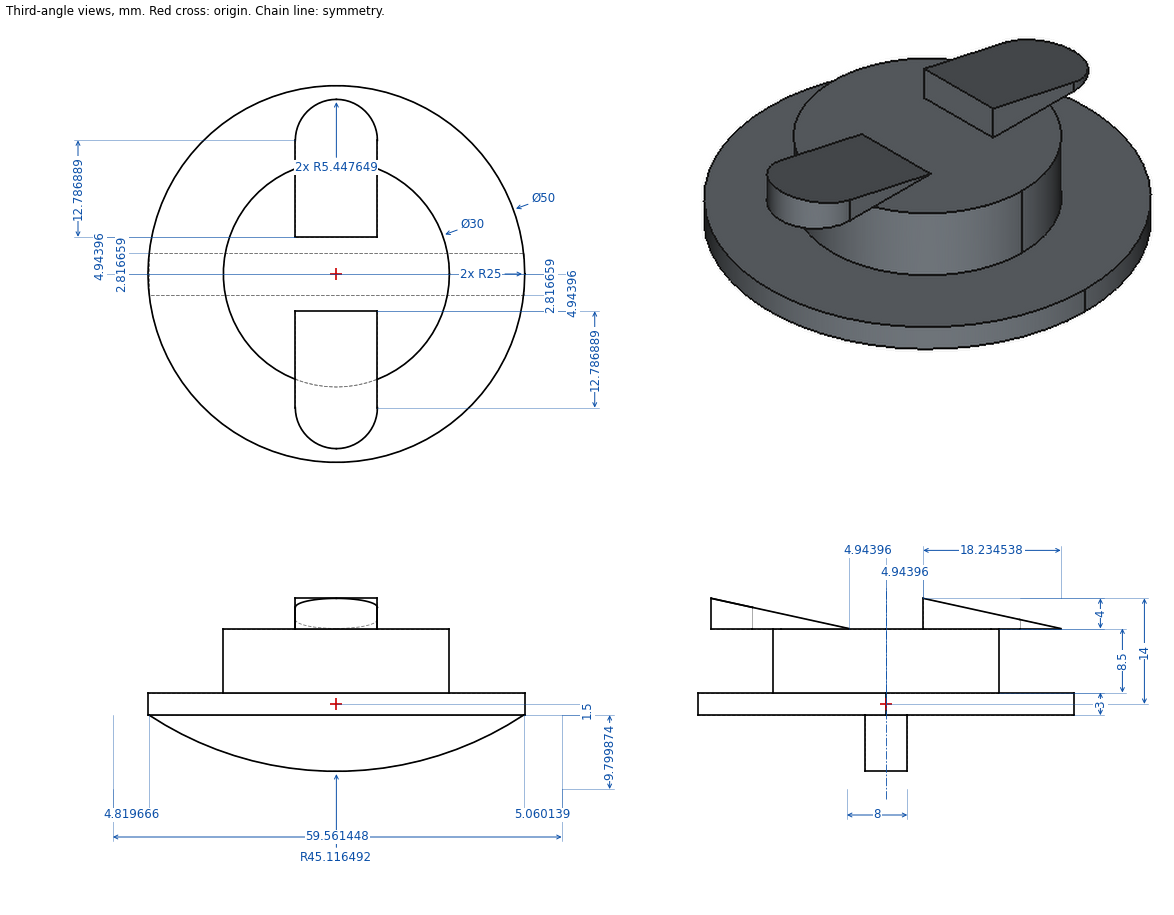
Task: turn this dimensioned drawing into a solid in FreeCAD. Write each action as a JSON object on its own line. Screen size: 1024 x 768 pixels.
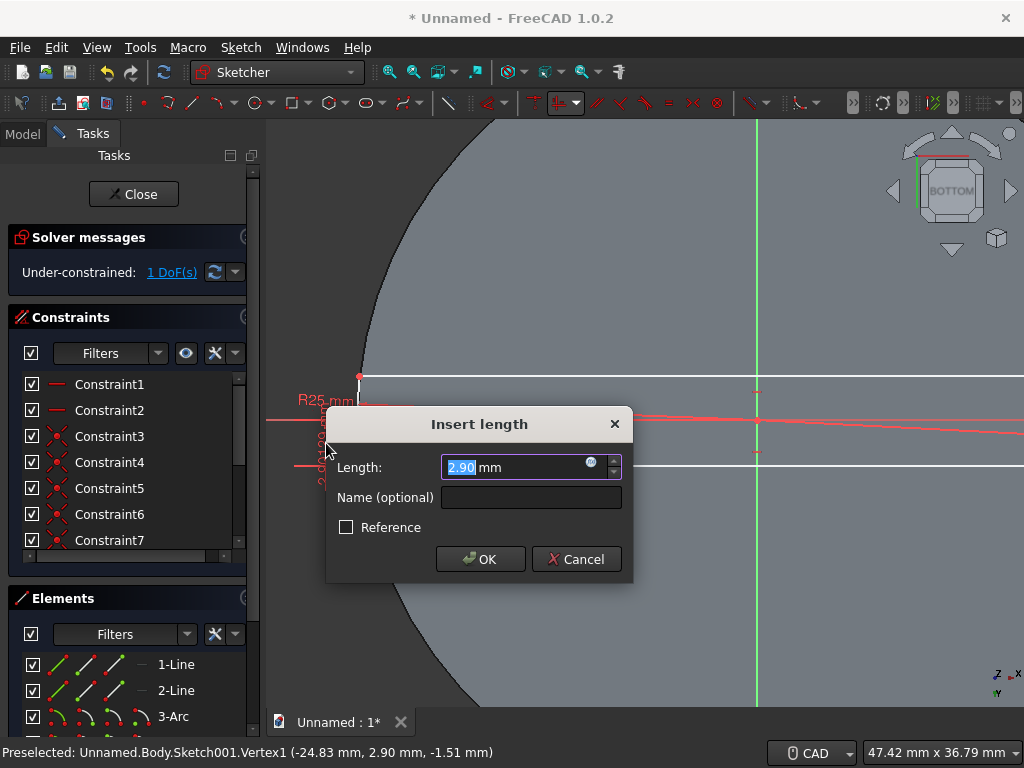
{"action": "type", "text": "2.816659"}
{"action": "key", "text": "Return"}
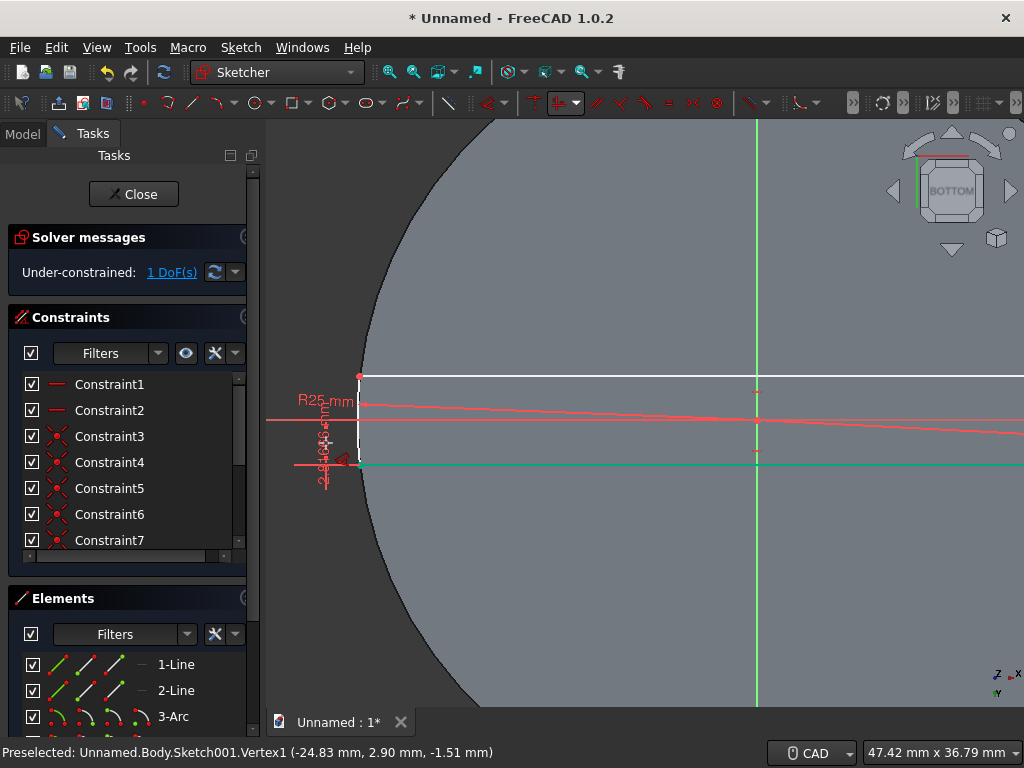
{"action": "scroll", "coordinate": [357, 404], "scroll_direction": "down", "scroll_amount": 3}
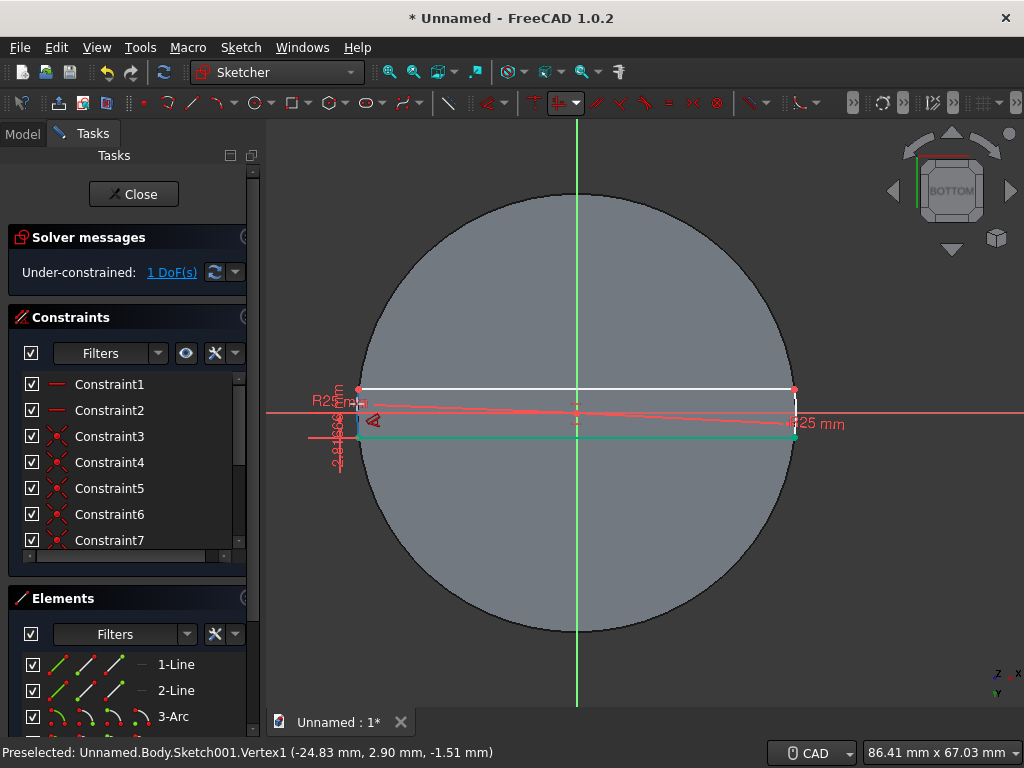
{"action": "scroll", "coordinate": [795, 389], "scroll_direction": "up", "scroll_amount": 3}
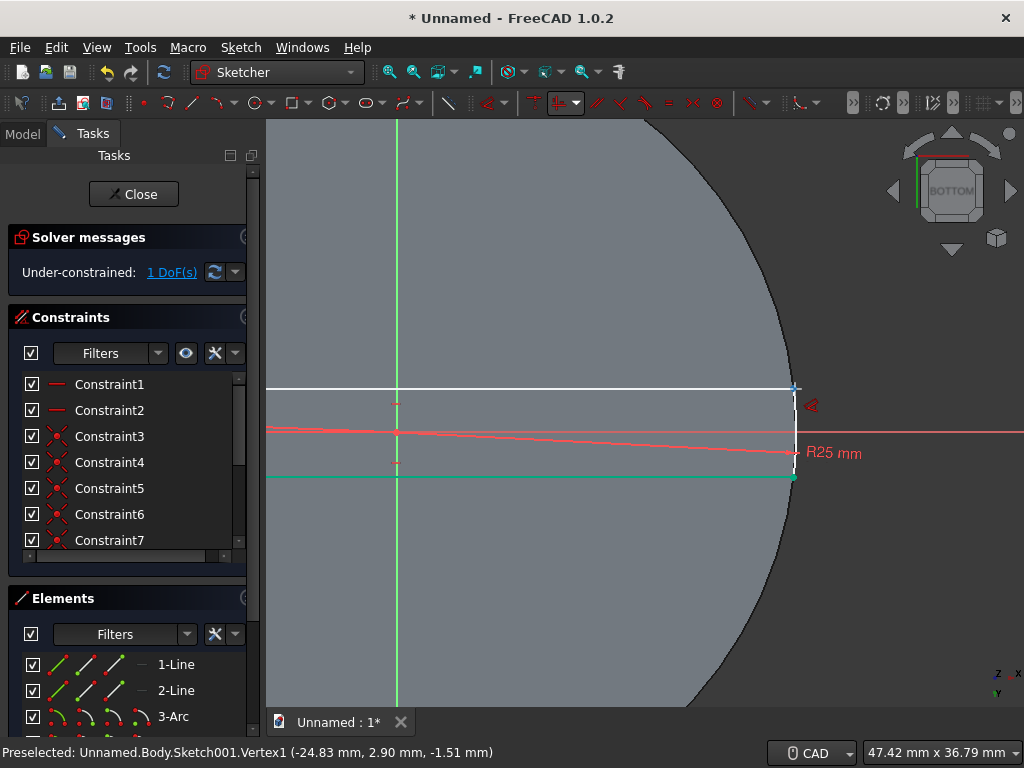
{"action": "left_click", "coordinate": [794, 389]}
{"action": "left_click", "coordinate": [828, 411]}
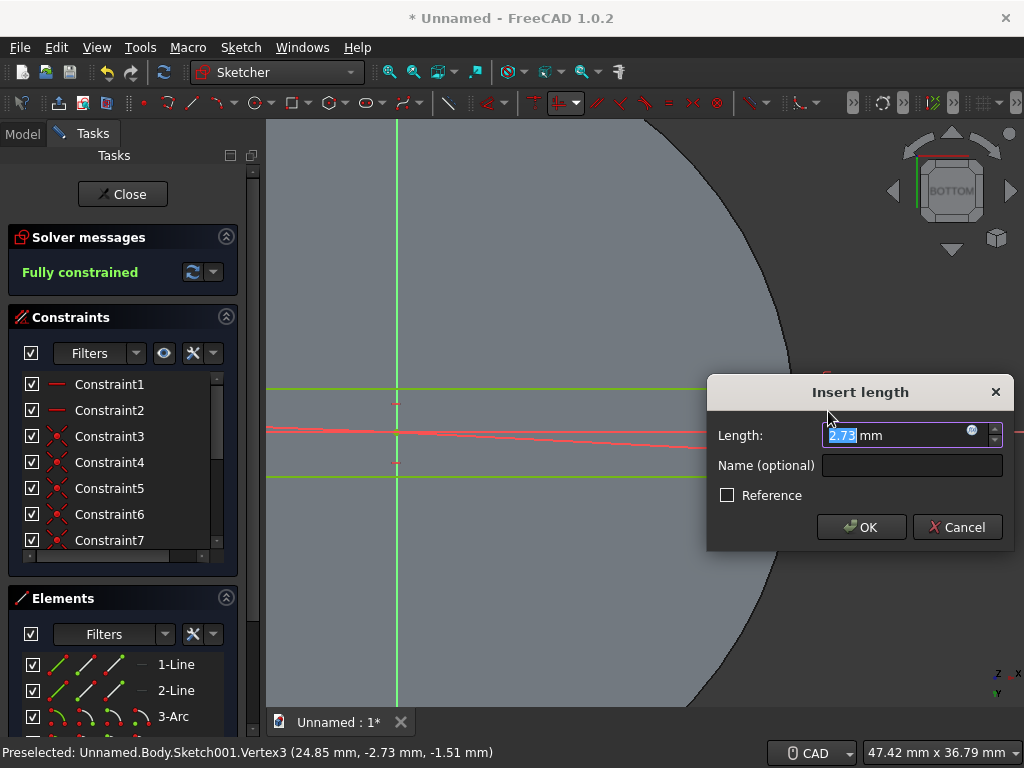
{"action": "type", "text": "2.816659"}
{"action": "key", "text": "Return"}
{"action": "key", "text": "Escape"}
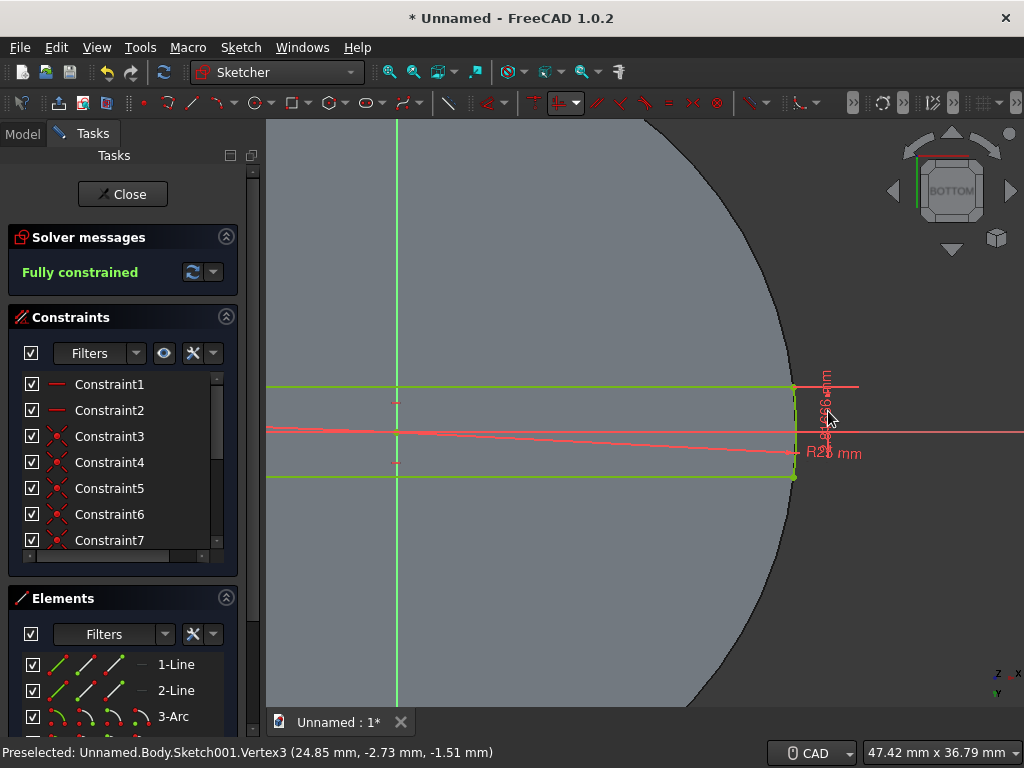
{"action": "left_click", "coordinate": [123, 194]}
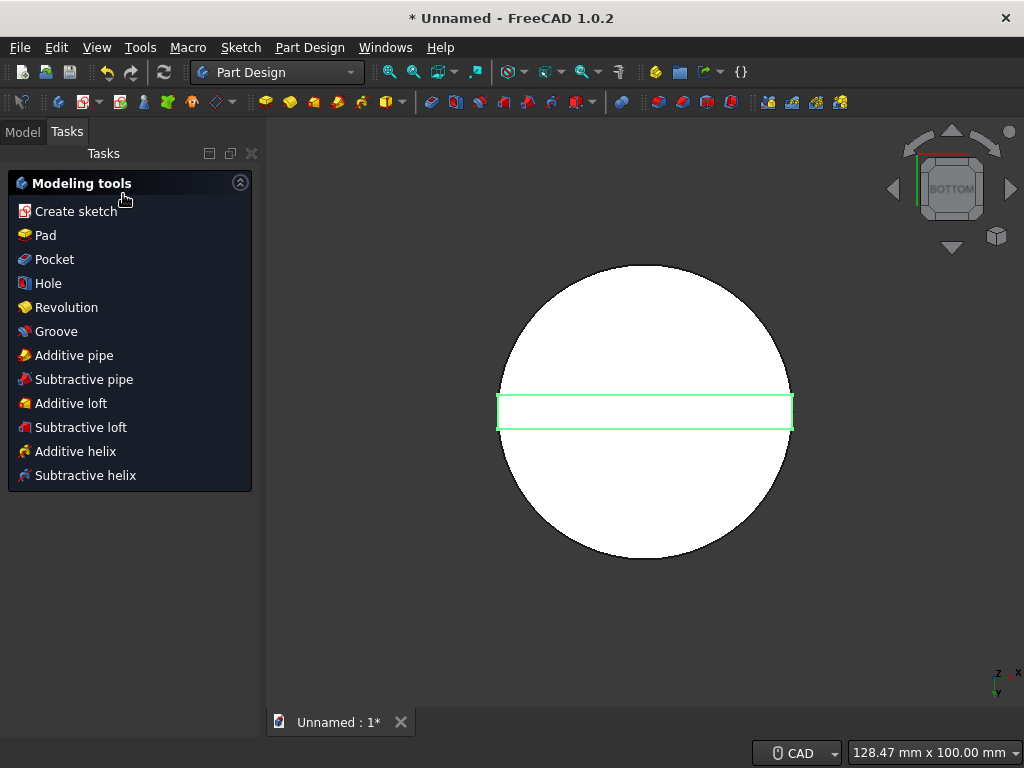
{"action": "left_click", "coordinate": [266, 102]}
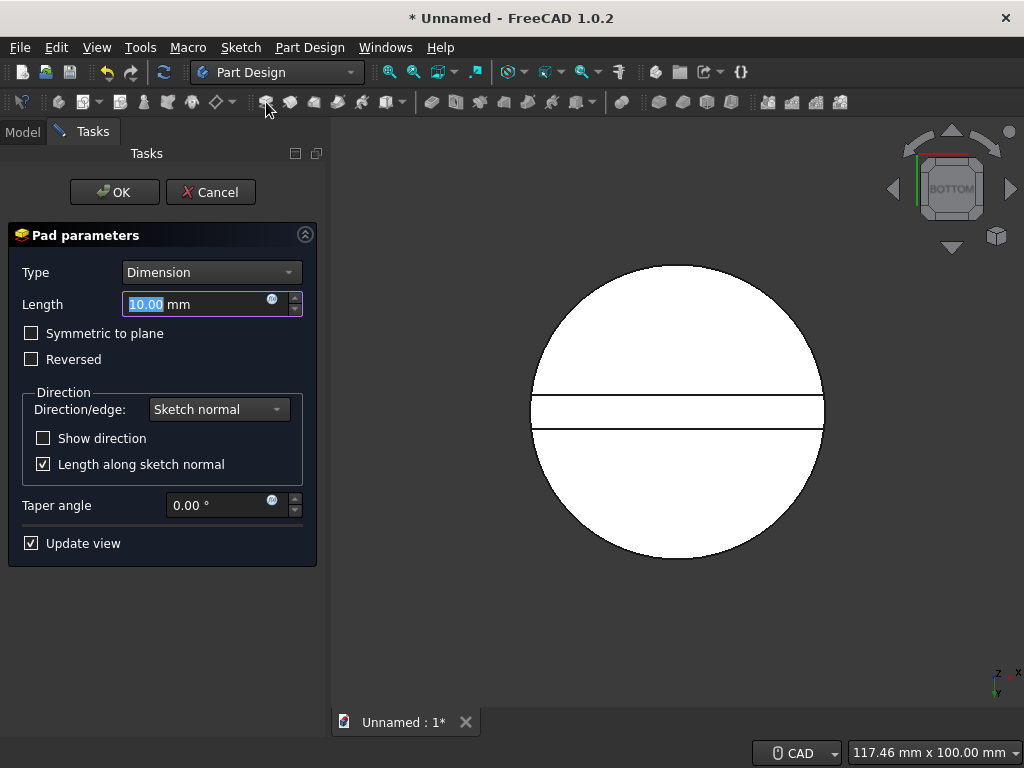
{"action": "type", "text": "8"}
{"action": "key", "text": "Tab"}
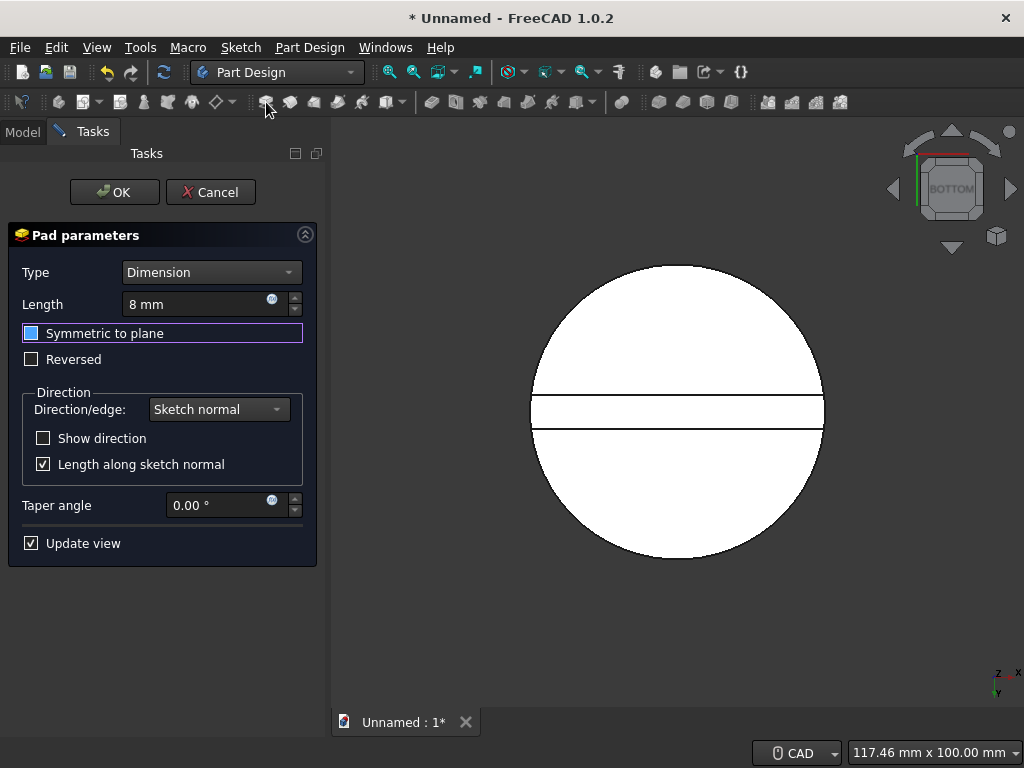
{"action": "left_click", "coordinate": [115, 192]}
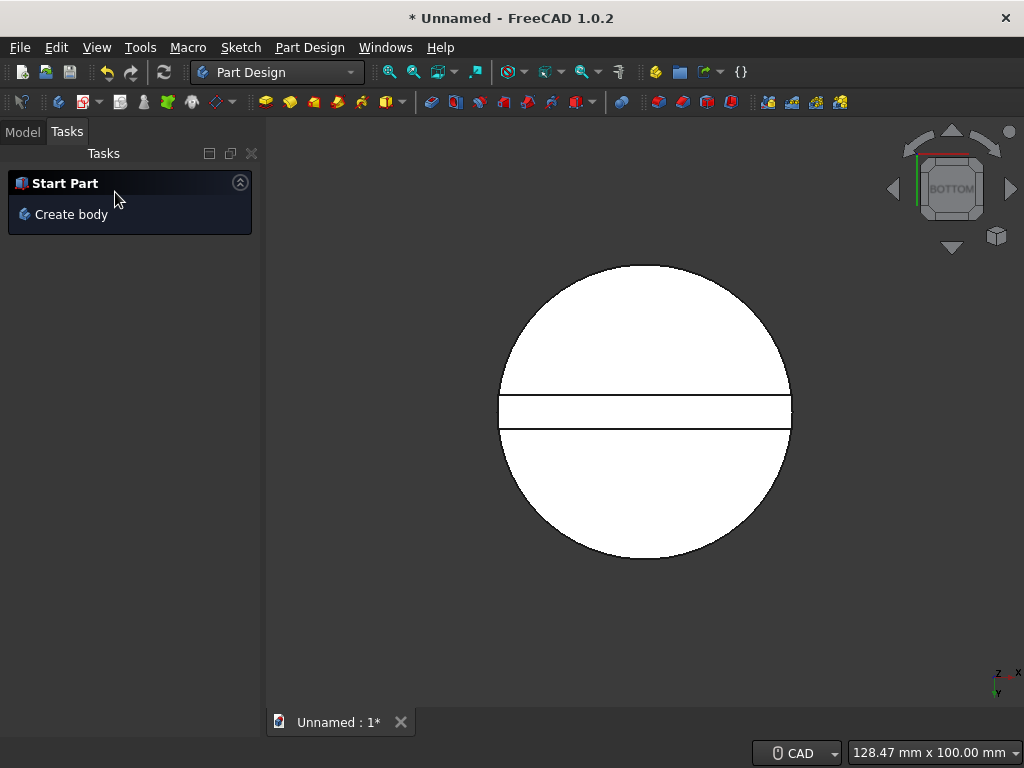
{"action": "key", "text": "4"}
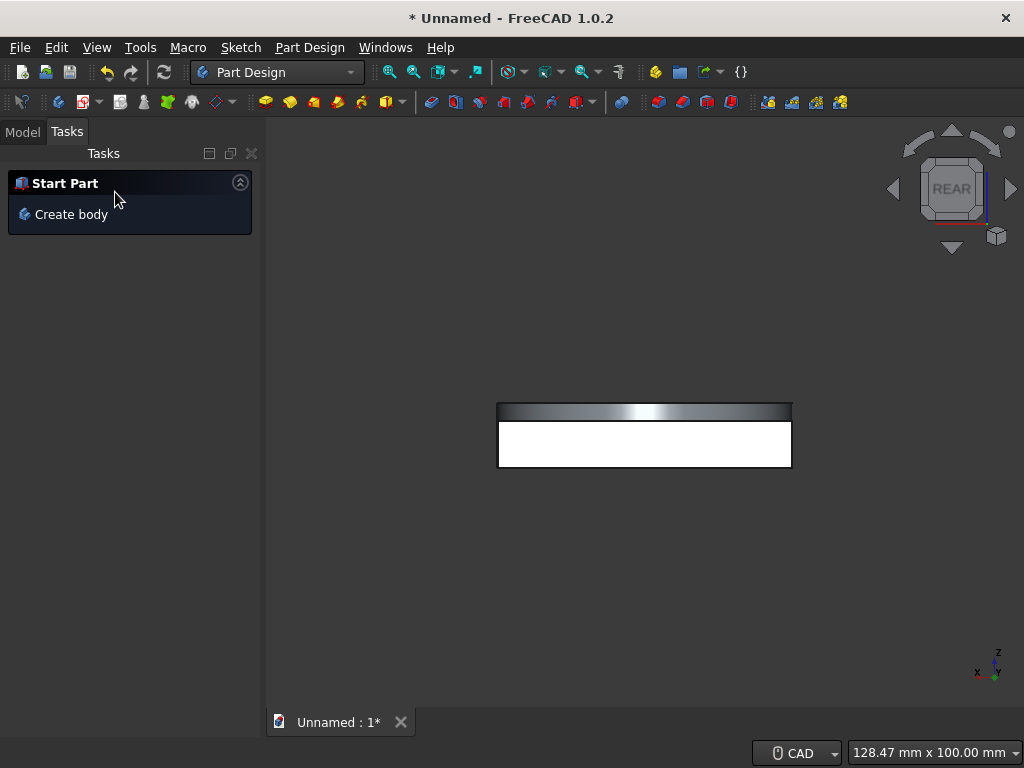
{"action": "left_click", "coordinate": [390, 72]}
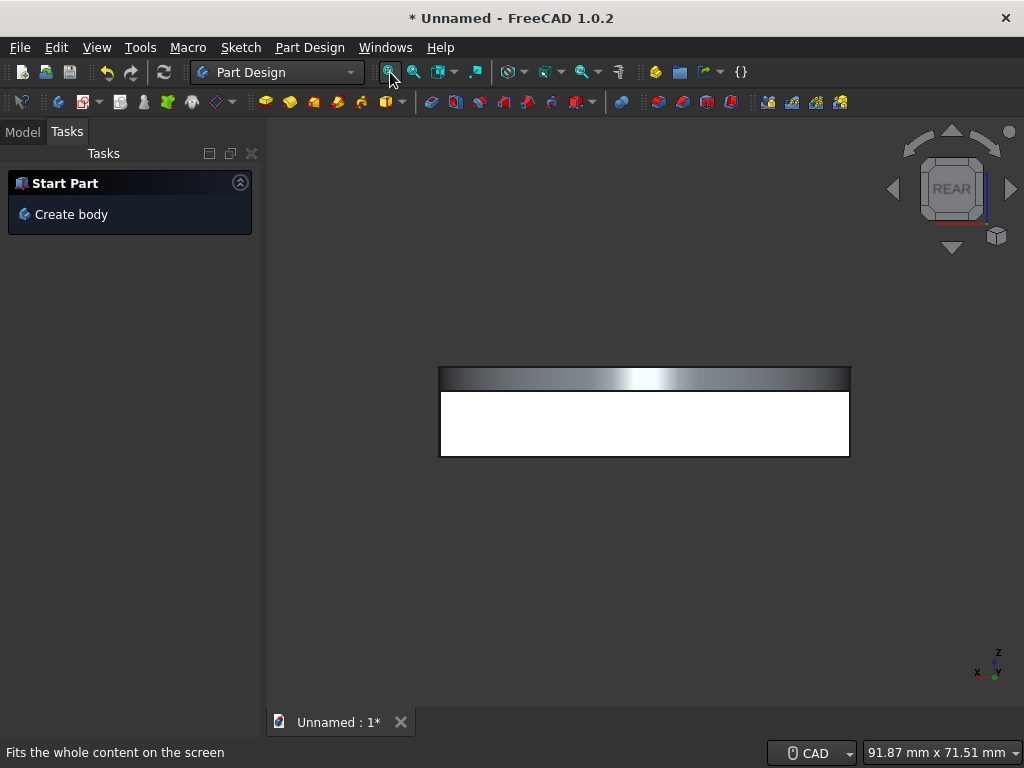
{"action": "left_click", "coordinate": [528, 423]}